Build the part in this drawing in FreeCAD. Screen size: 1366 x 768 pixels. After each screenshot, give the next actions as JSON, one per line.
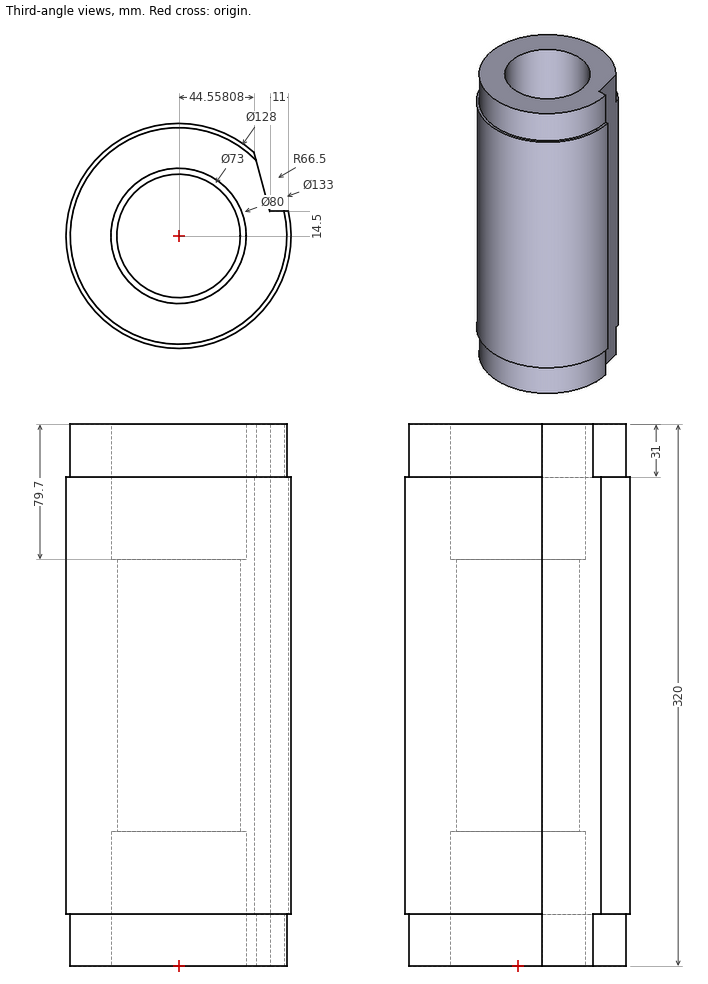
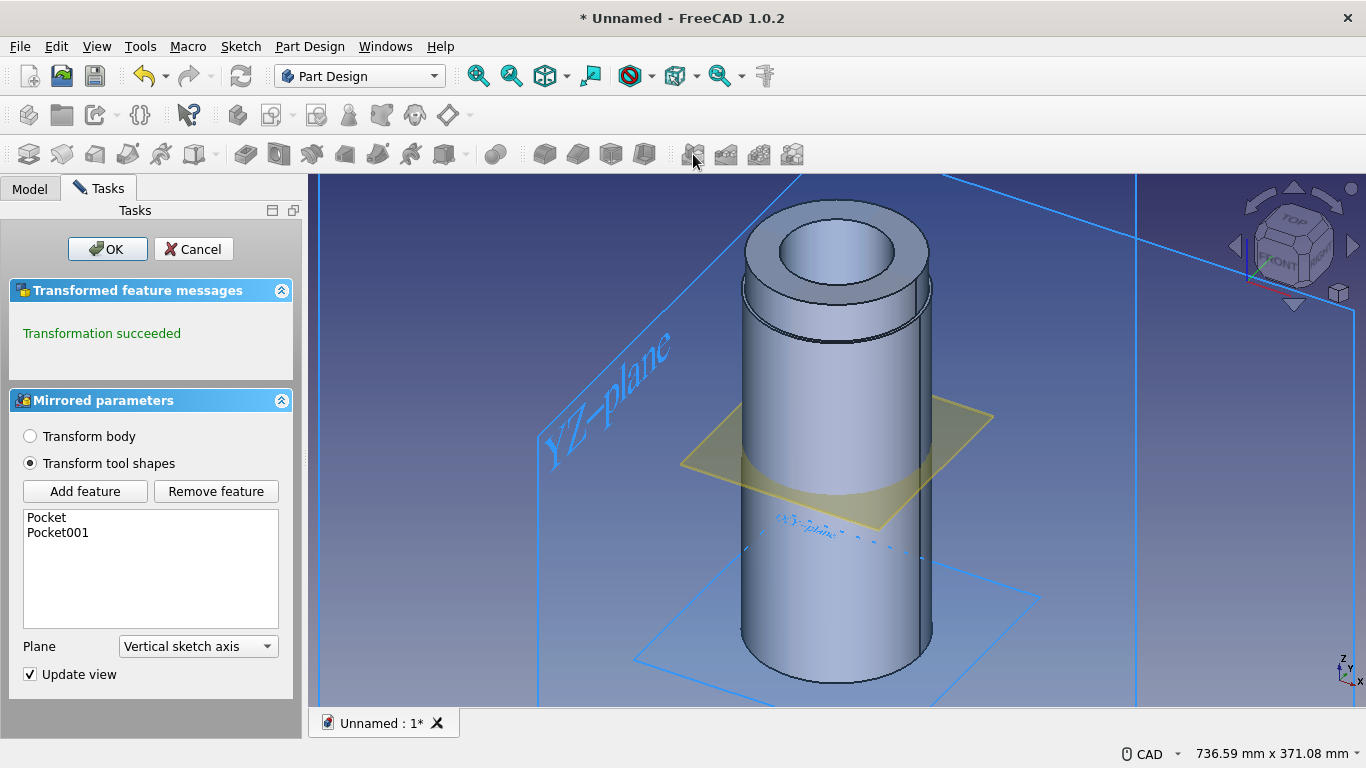
{"action": "left_click", "coordinate": [199, 646]}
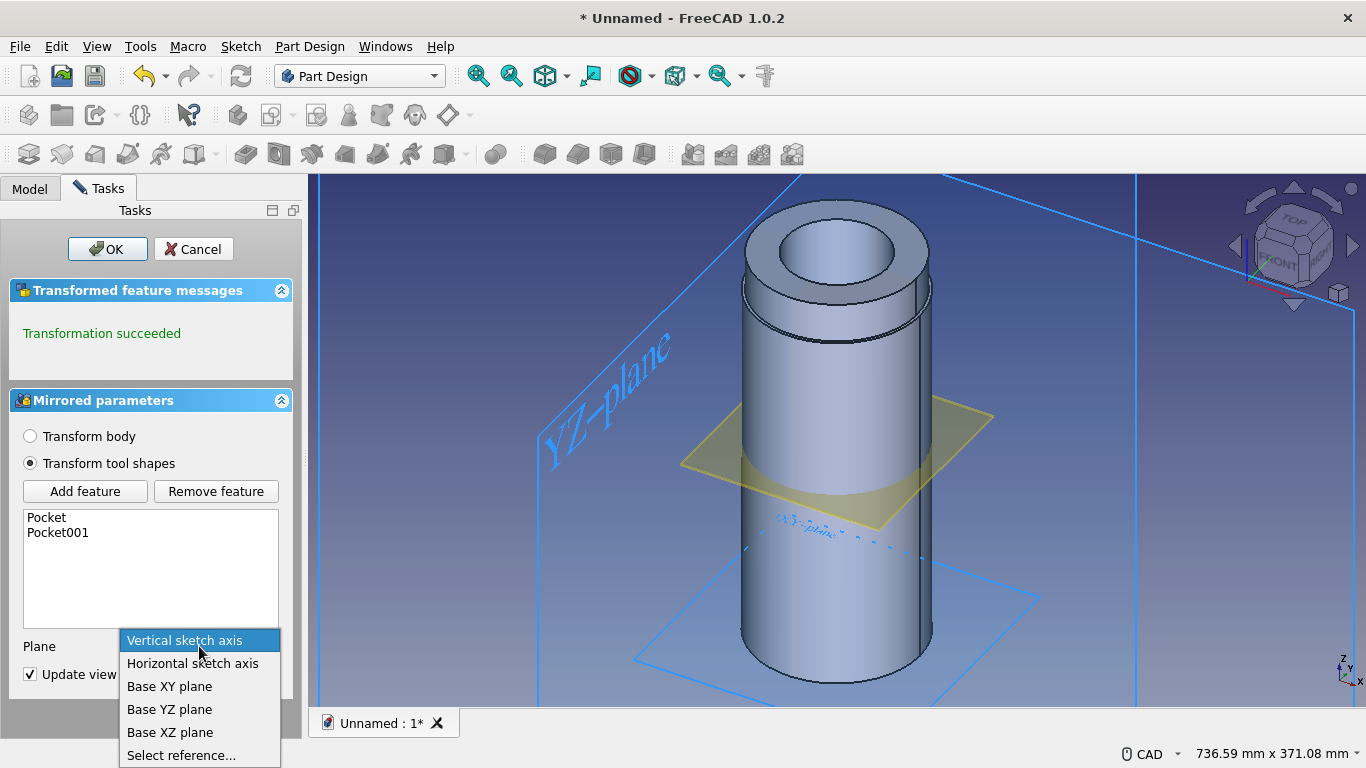
{"action": "left_click", "coordinate": [198, 756]}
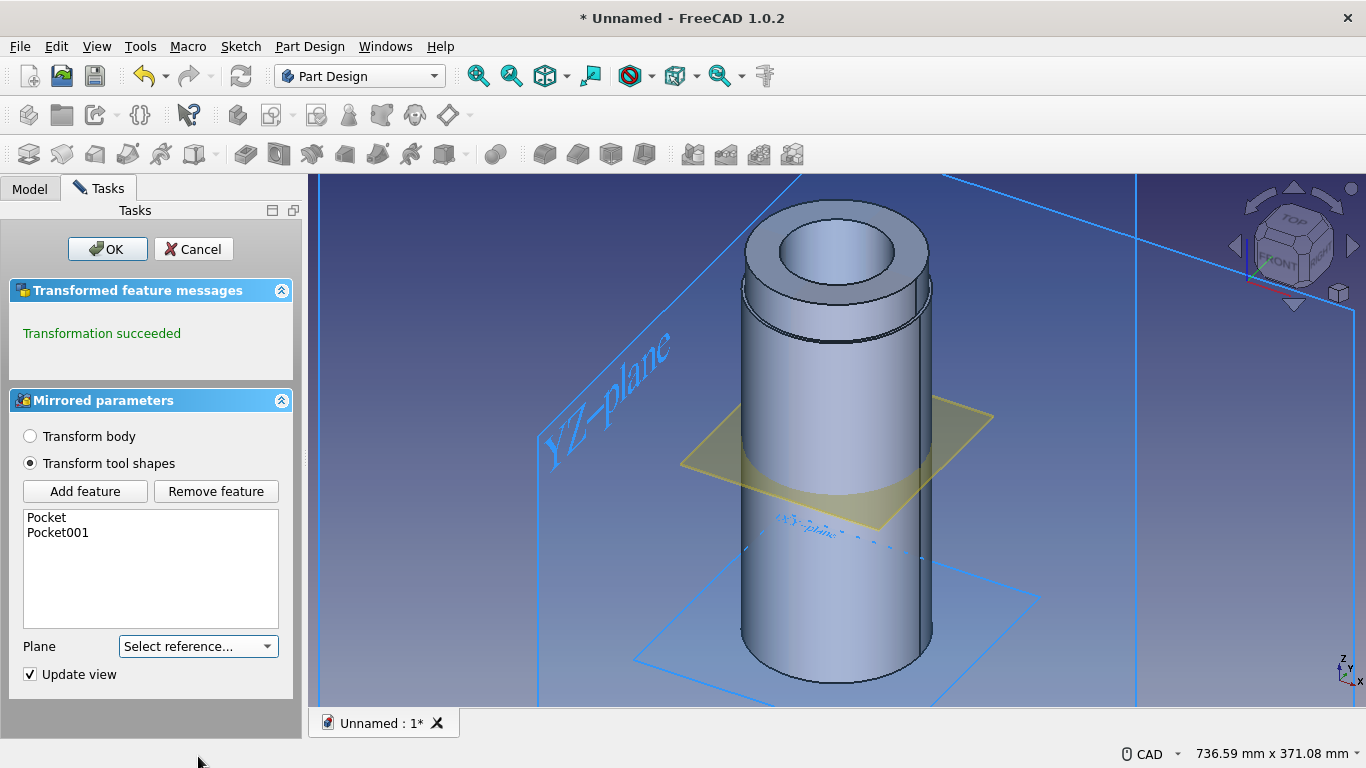
{"action": "left_click", "coordinate": [30, 188]}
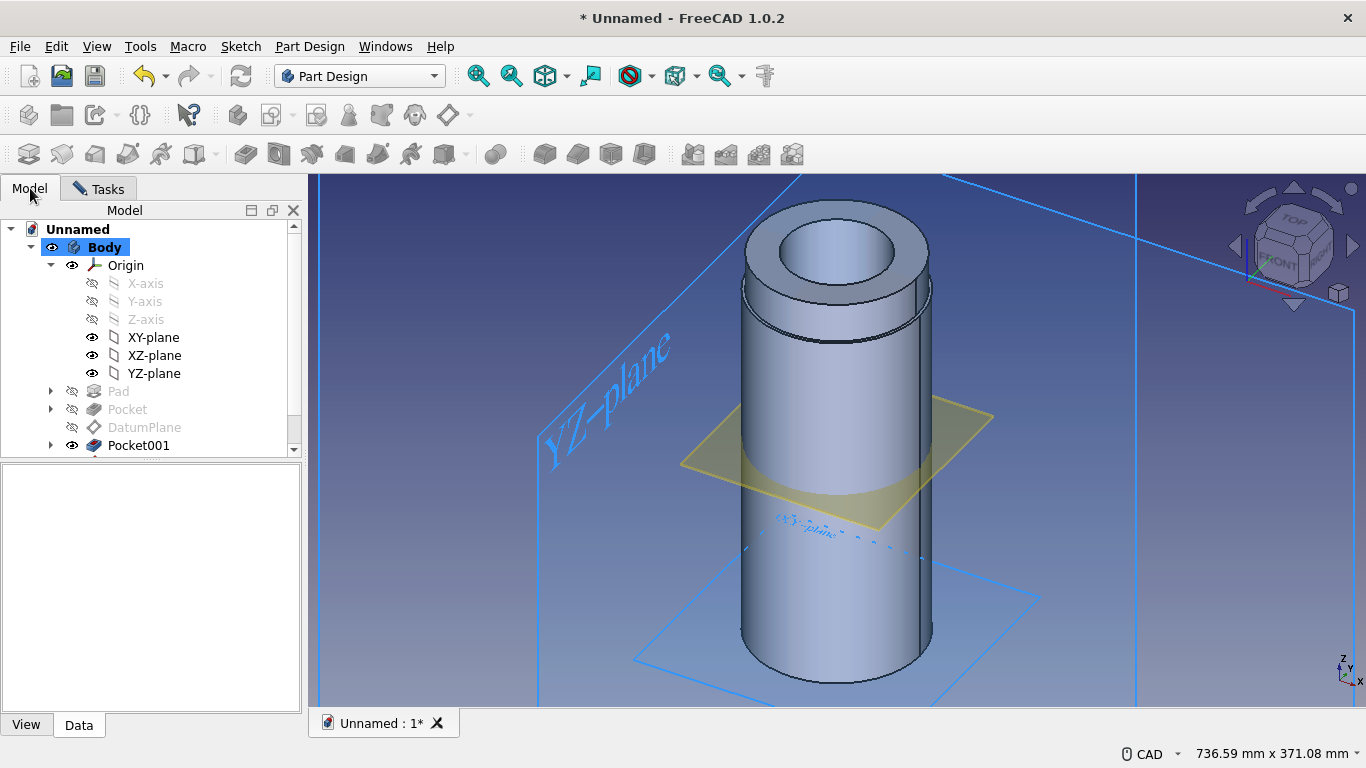
{"action": "scroll", "coordinate": [101, 333], "scroll_direction": "down", "scroll_amount": 3}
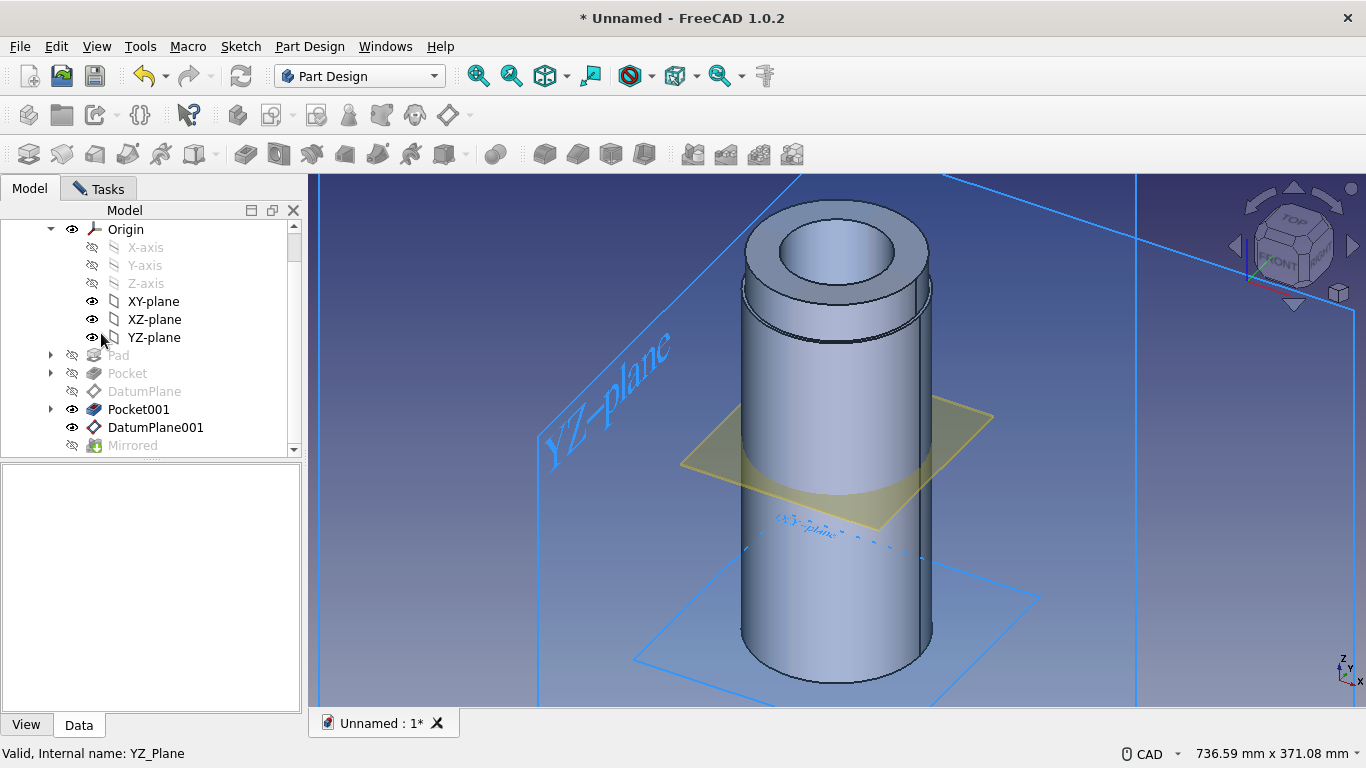
{"action": "left_click", "coordinate": [117, 427]}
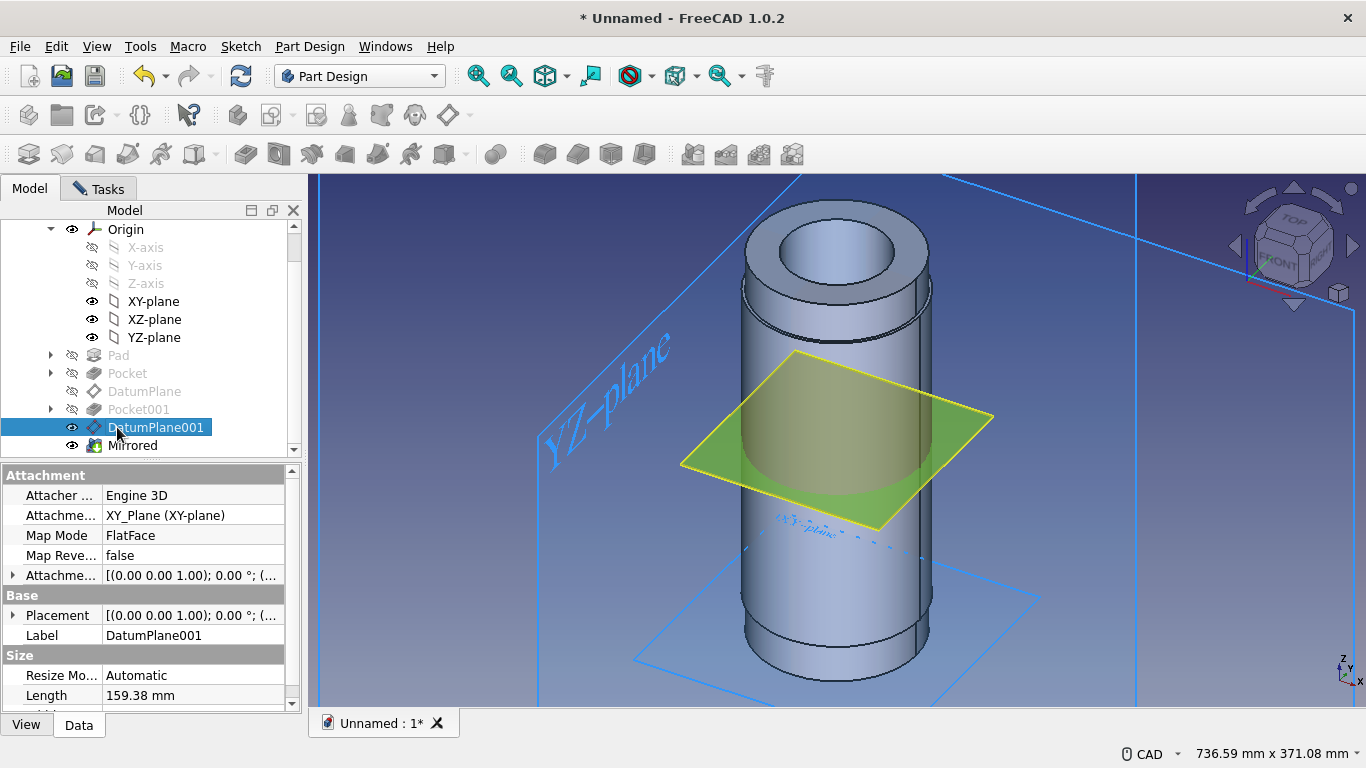
{"action": "left_click", "coordinate": [98, 188]}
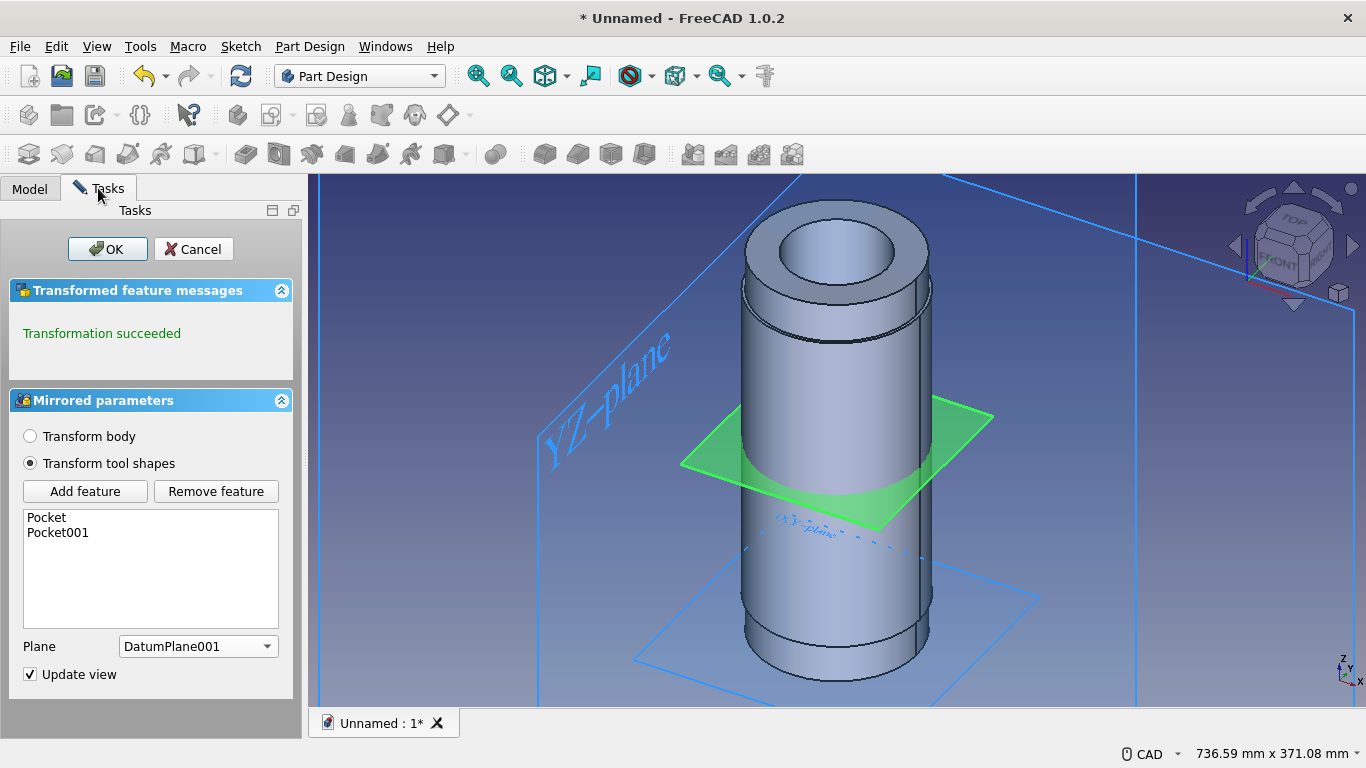
{"action": "left_click", "coordinate": [108, 249]}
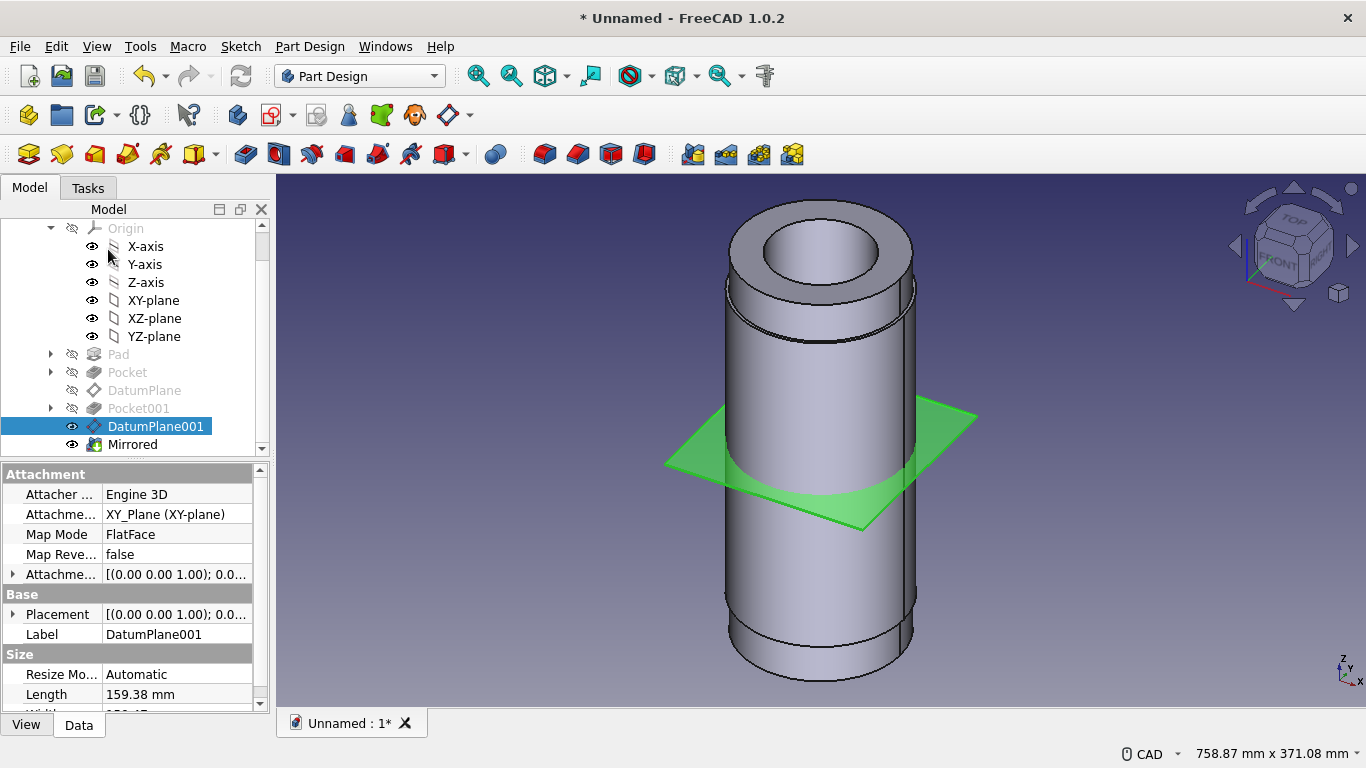
{"action": "left_click", "coordinate": [117, 426]}
{"action": "key", "text": "space"}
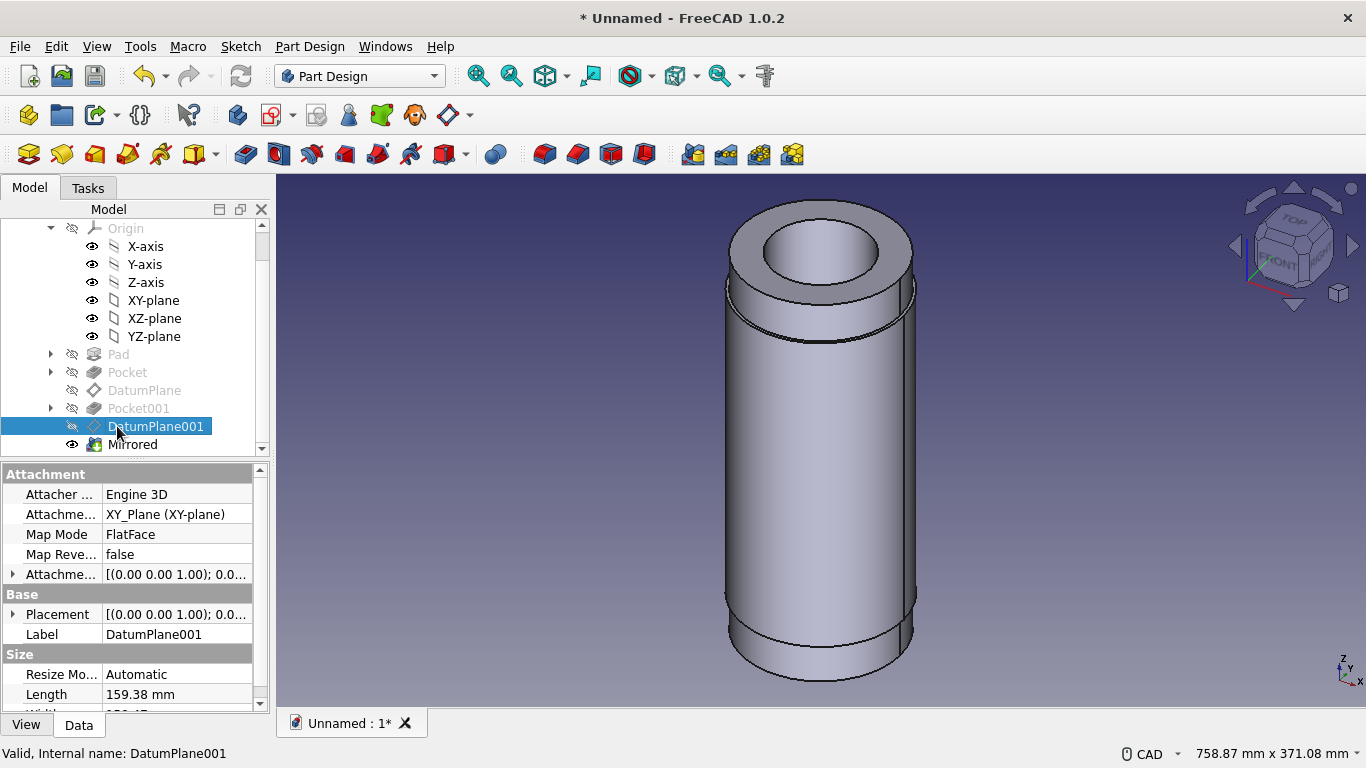
{"action": "left_click", "coordinate": [893, 240]}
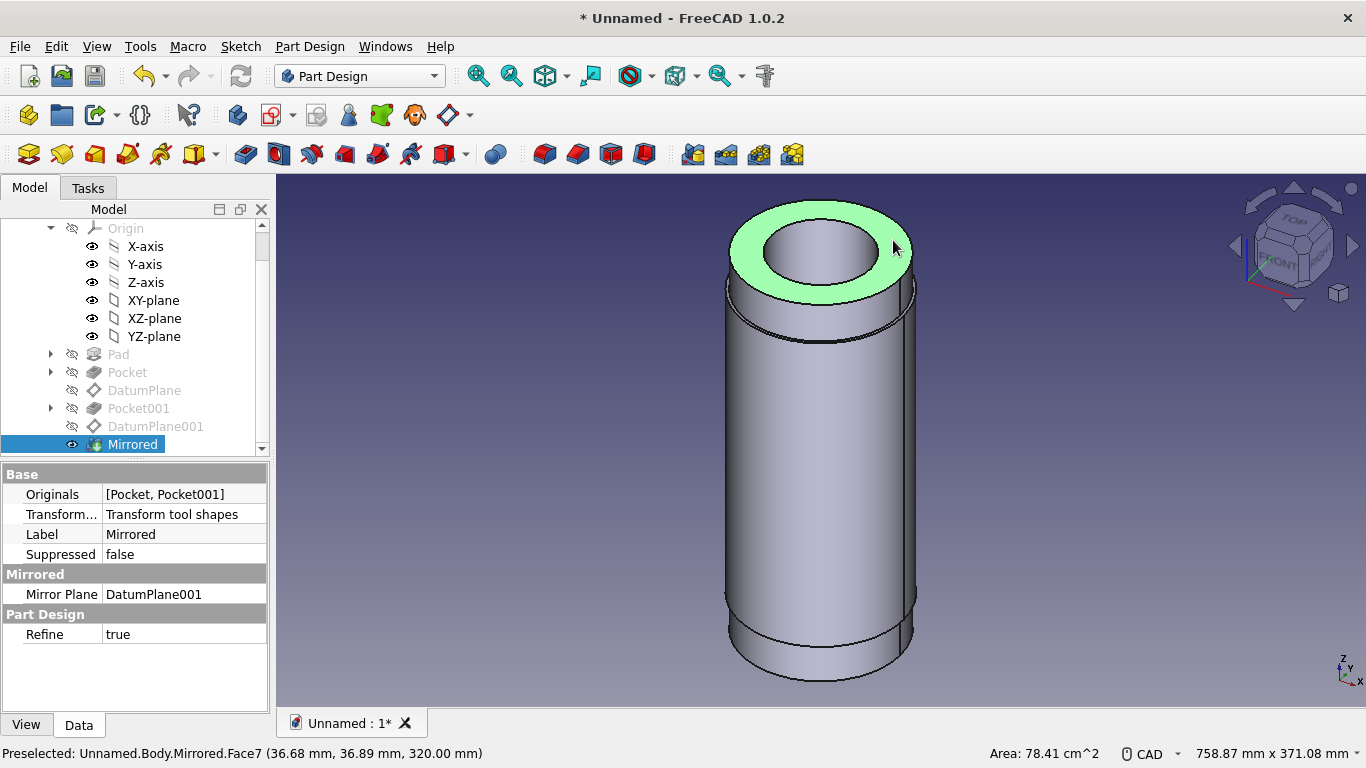
{"action": "left_click", "coordinate": [270, 116]}